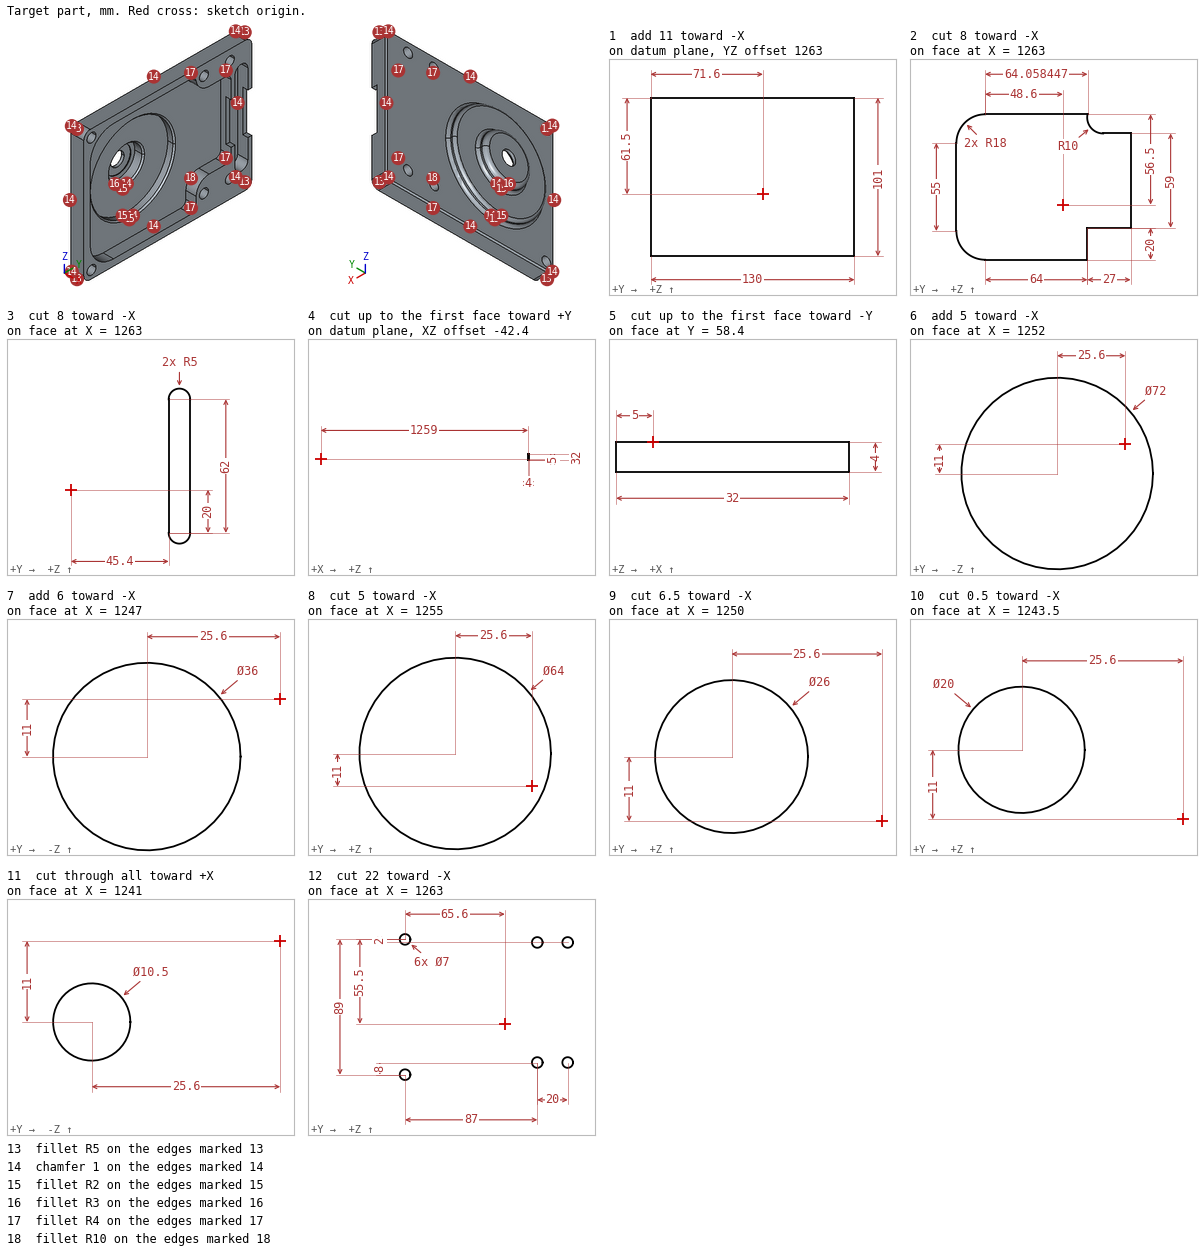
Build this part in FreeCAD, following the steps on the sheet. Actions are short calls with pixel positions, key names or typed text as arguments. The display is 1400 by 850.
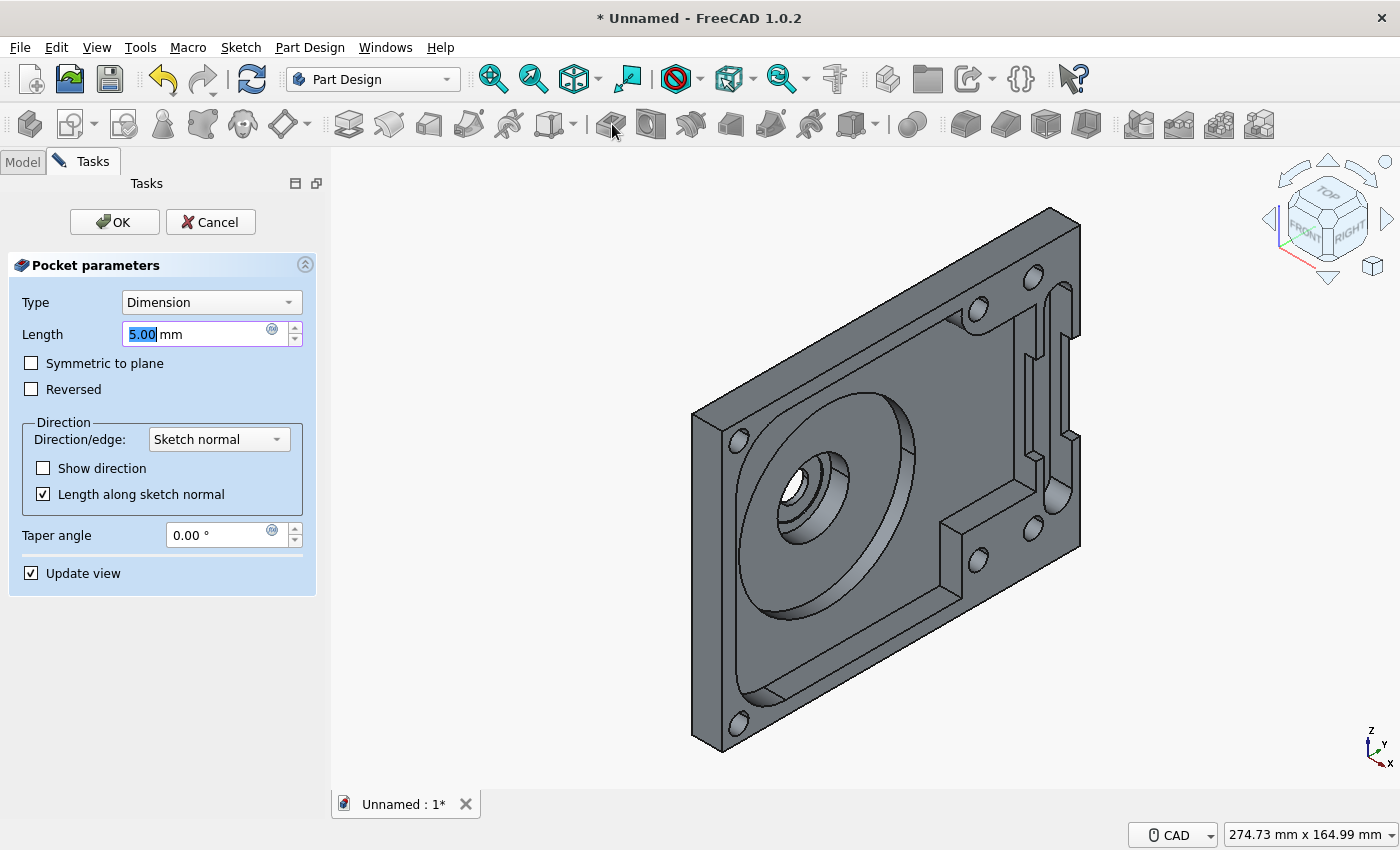
text(22)
key(Tab)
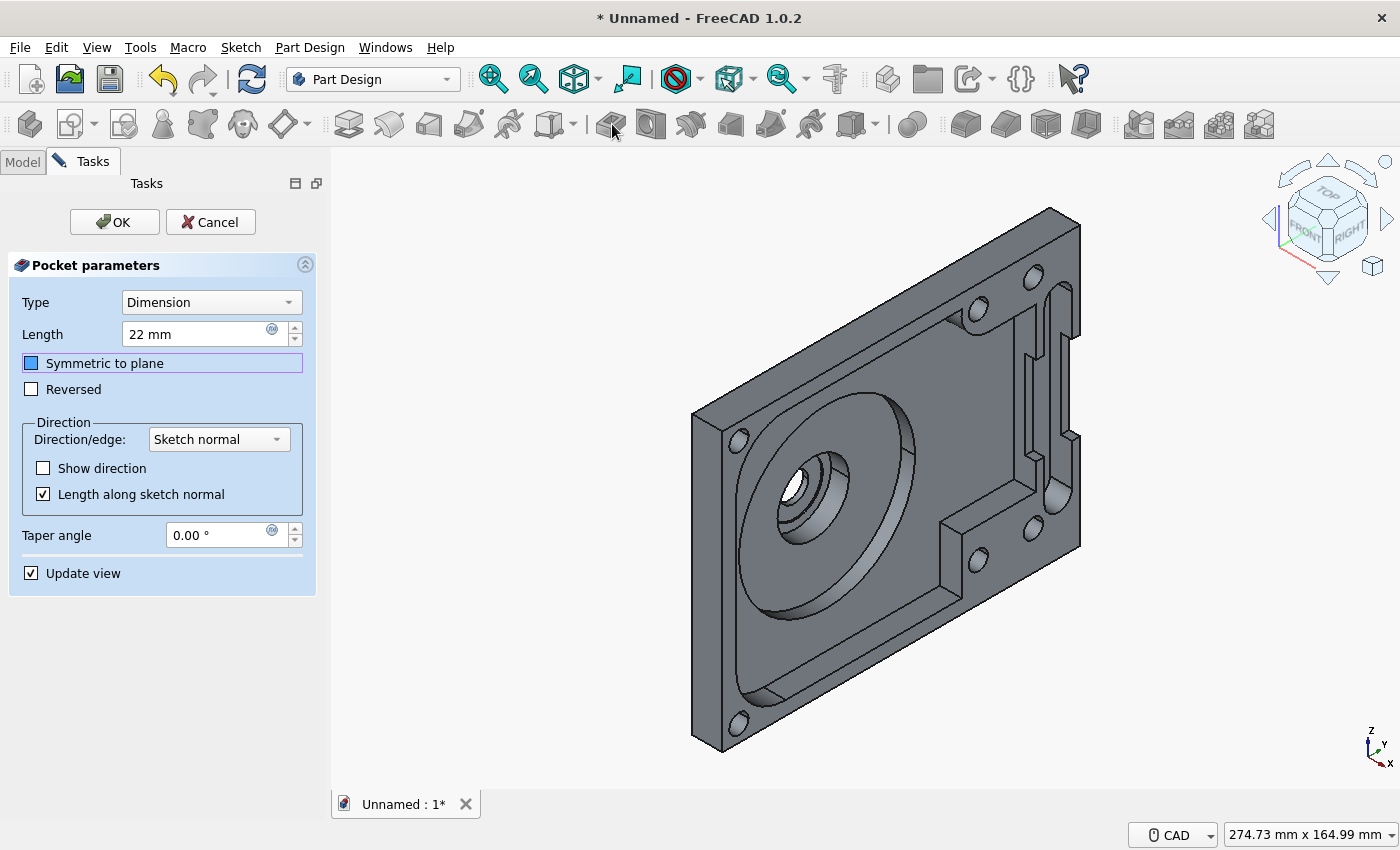
click(115, 222)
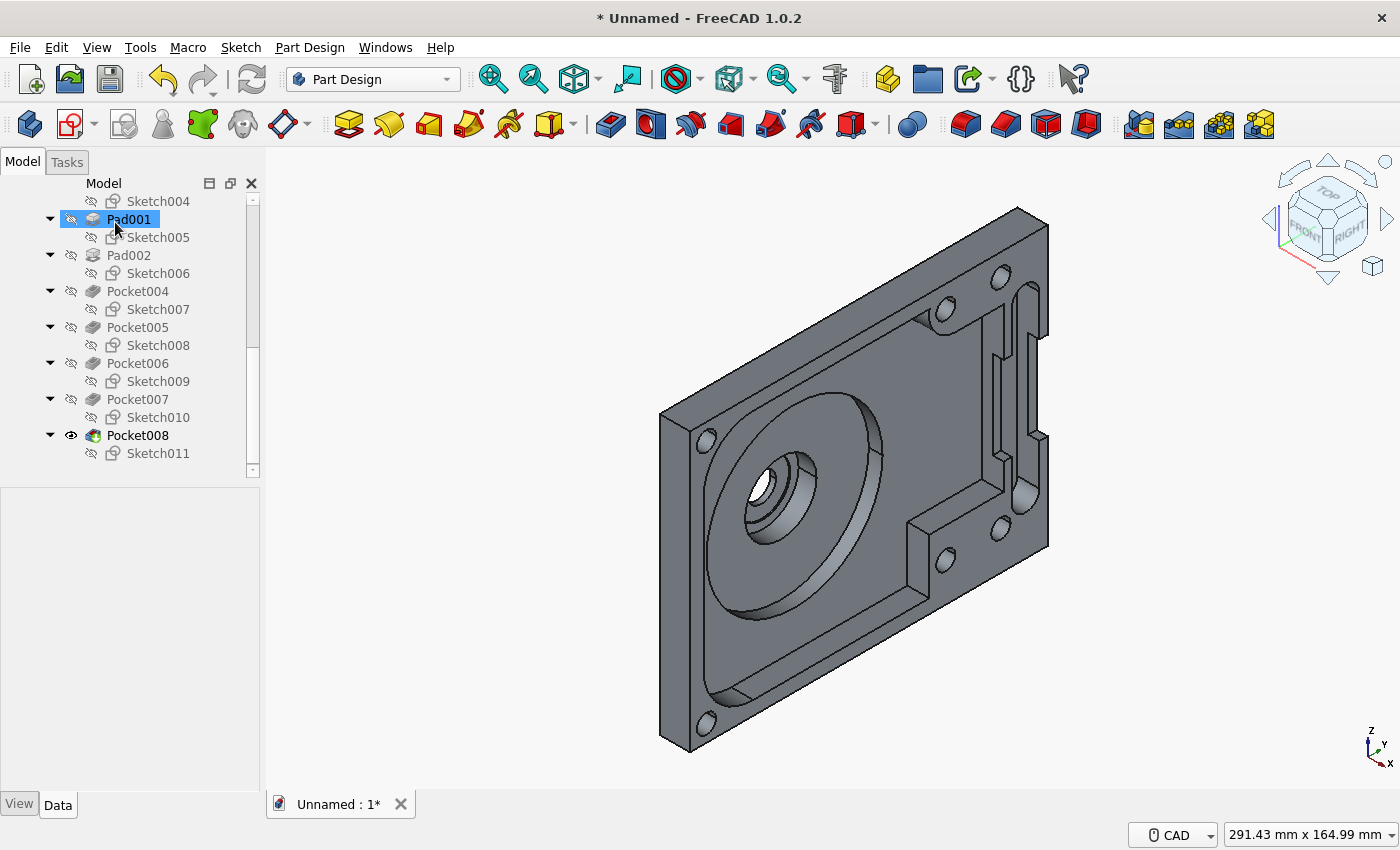
click(675, 422)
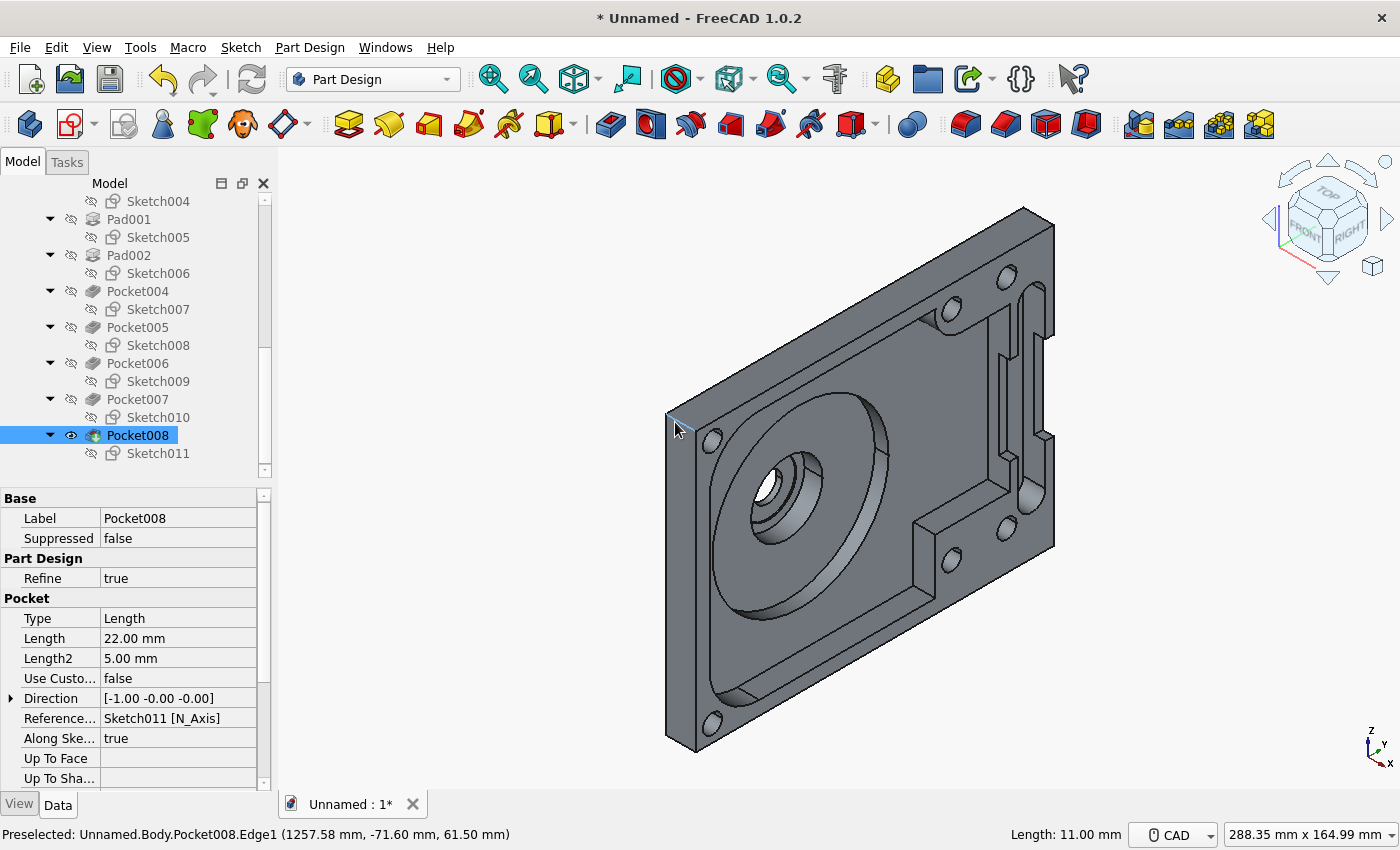
key(2)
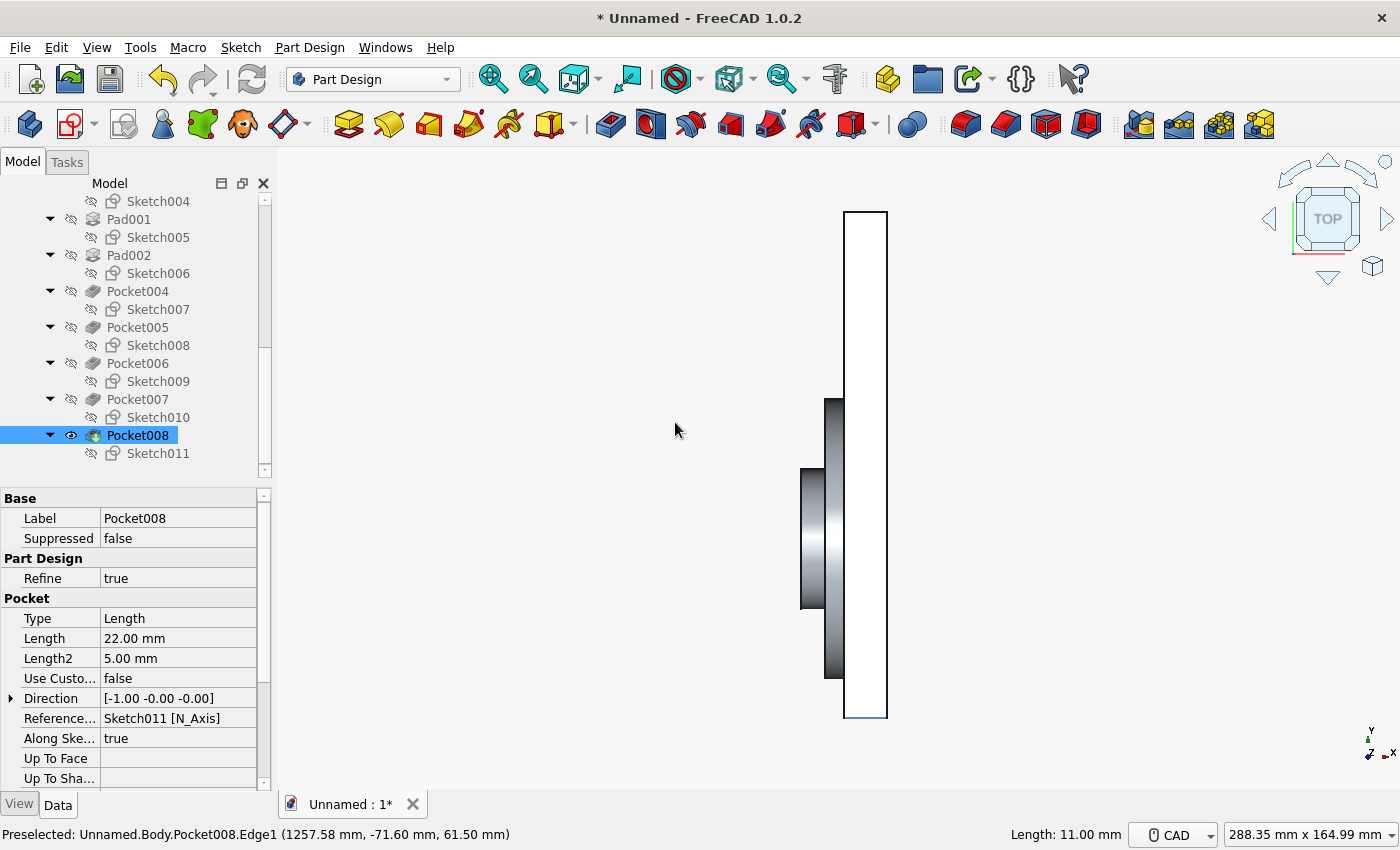
click(866, 211, ctrl)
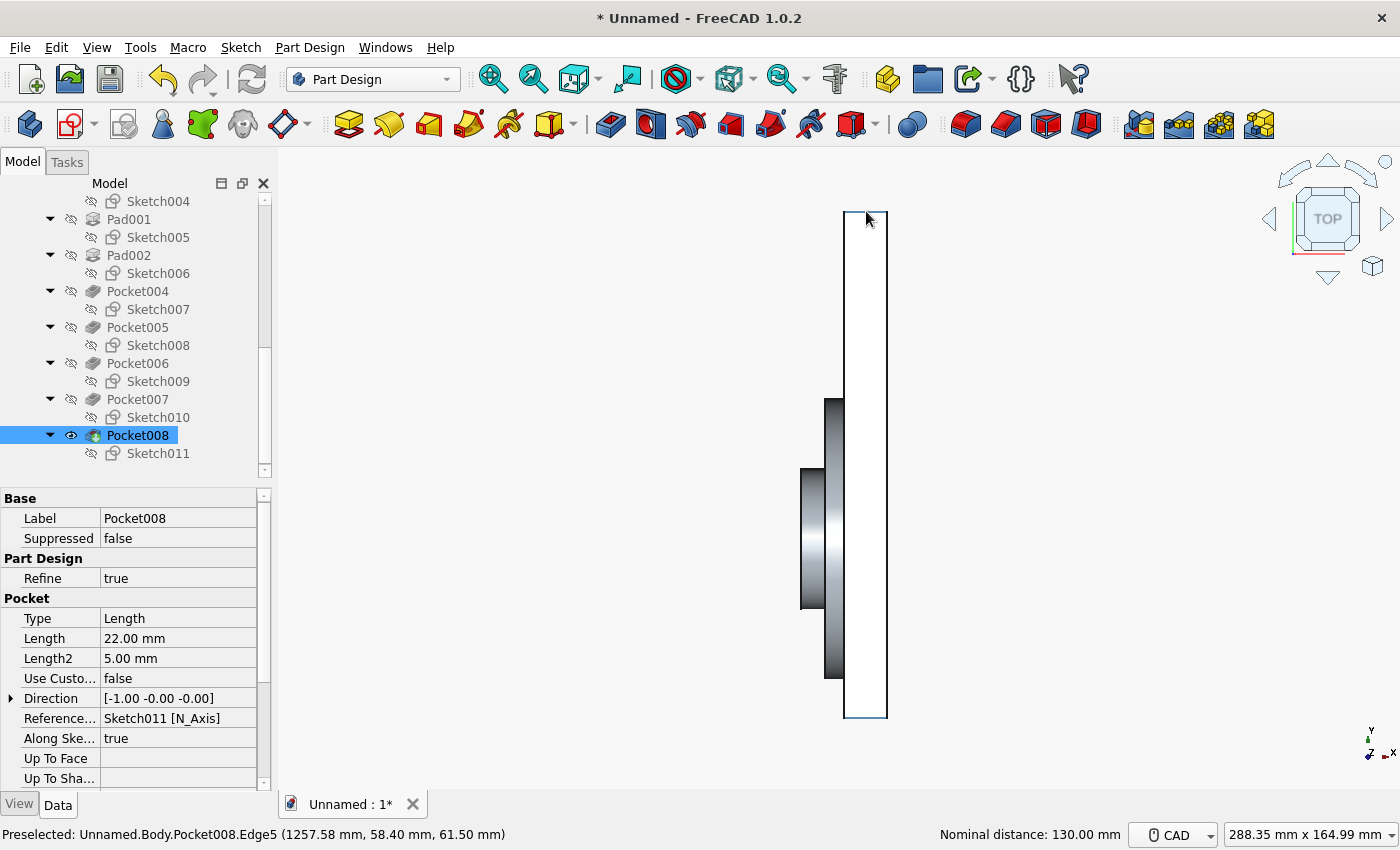
key(0)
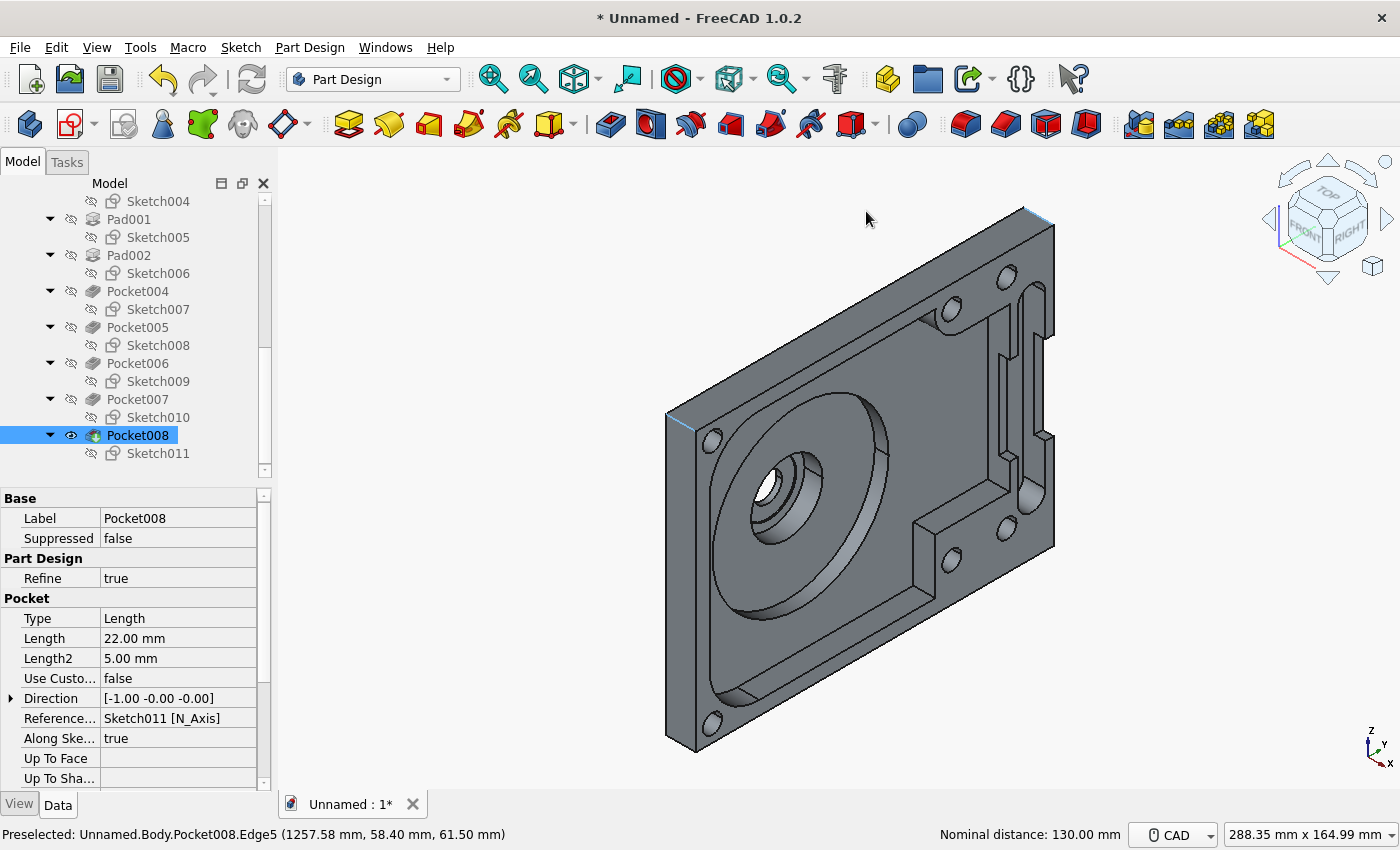
key(1)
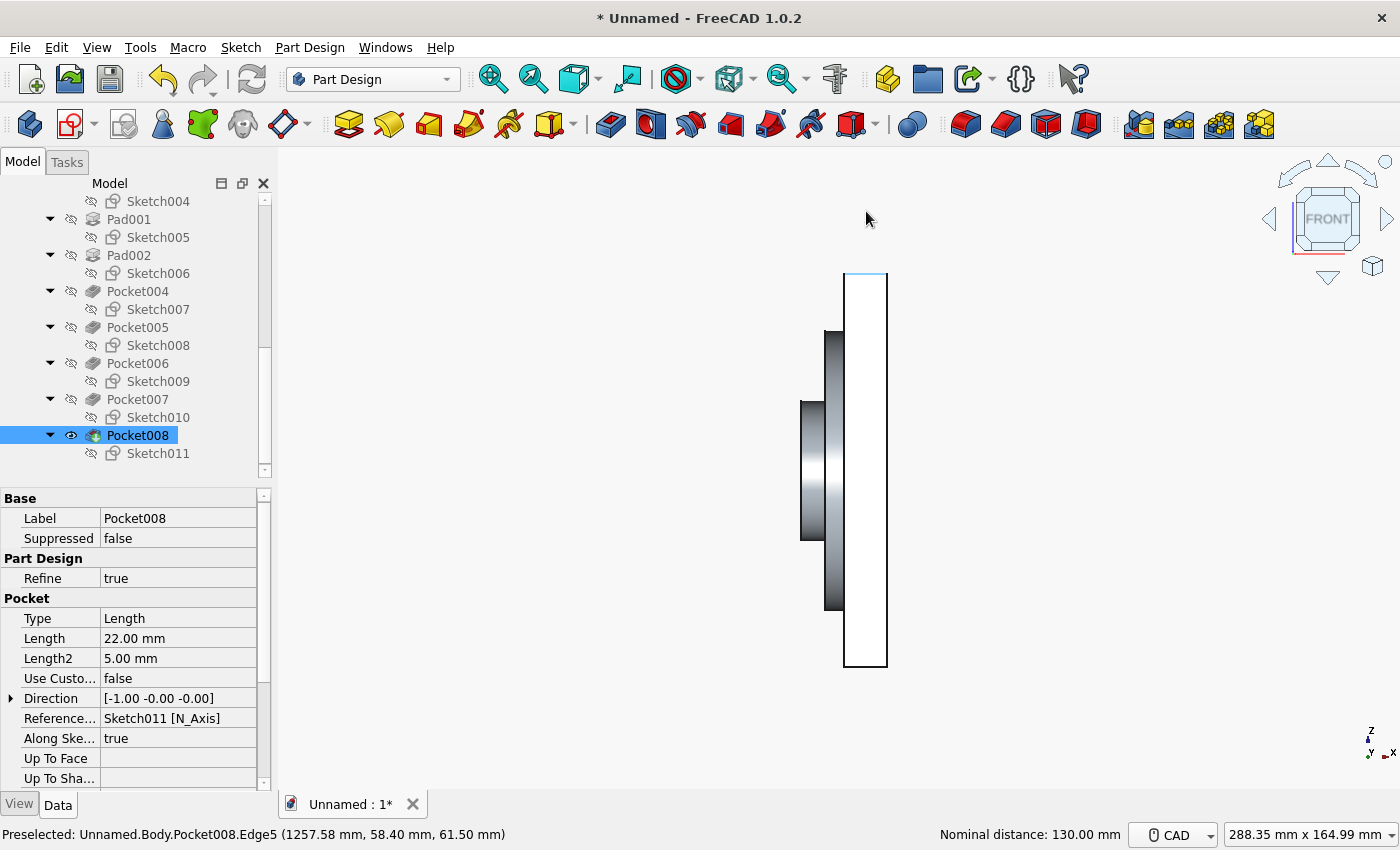
click(866, 666, ctrl)